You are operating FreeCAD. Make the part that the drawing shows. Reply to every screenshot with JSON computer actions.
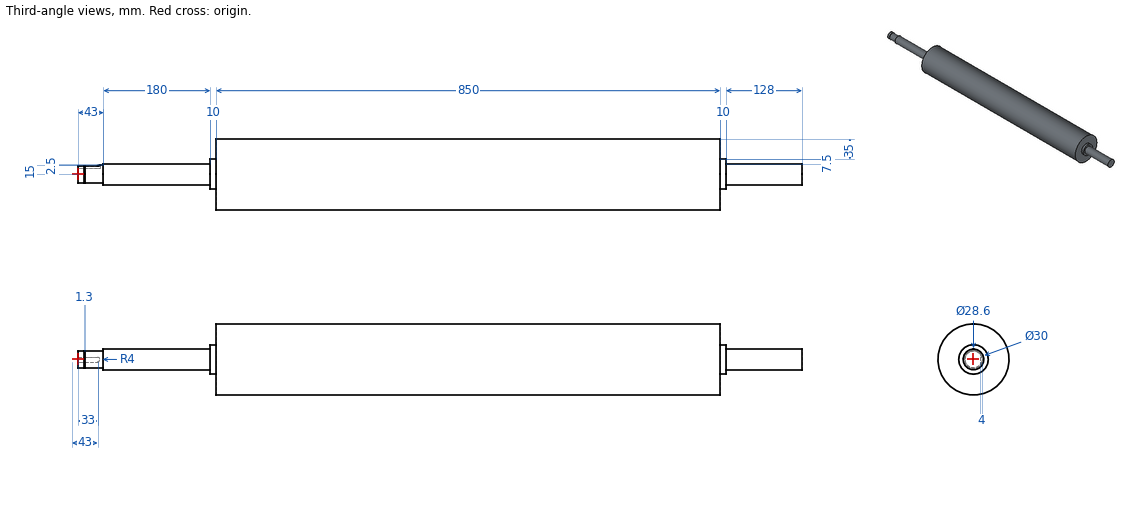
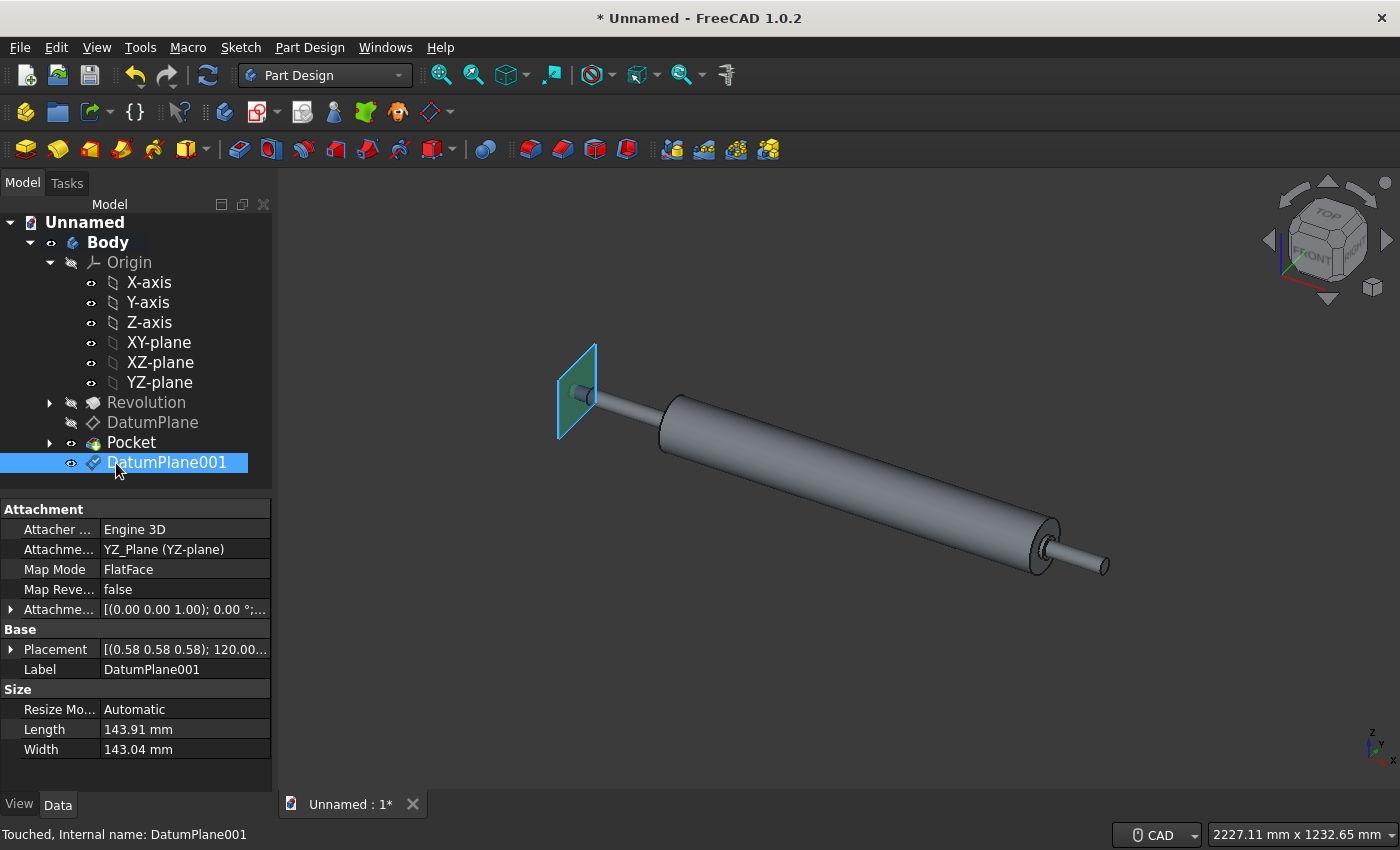
{"action": "left_click", "coordinate": [258, 112]}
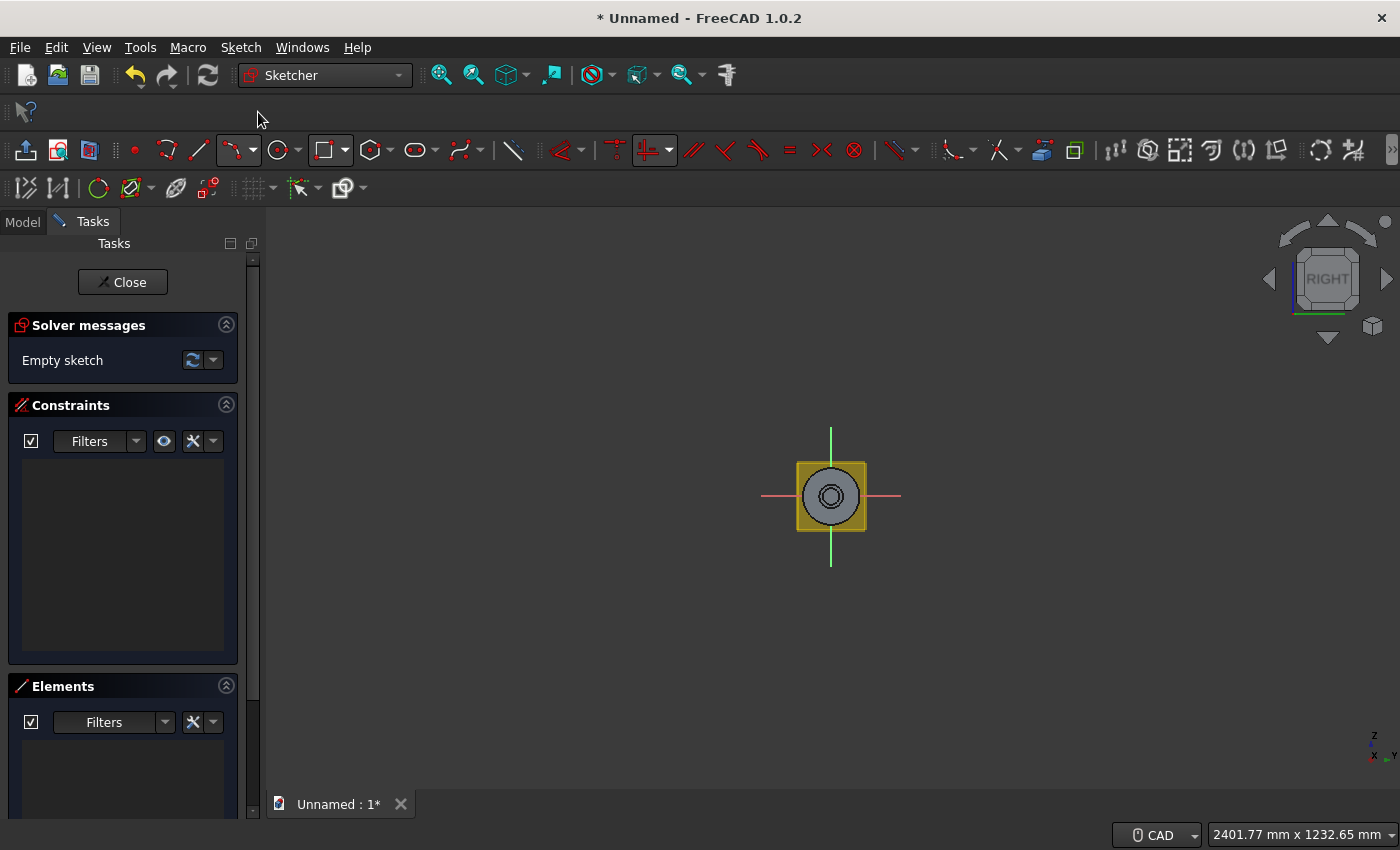
{"action": "left_click", "coordinate": [90, 150]}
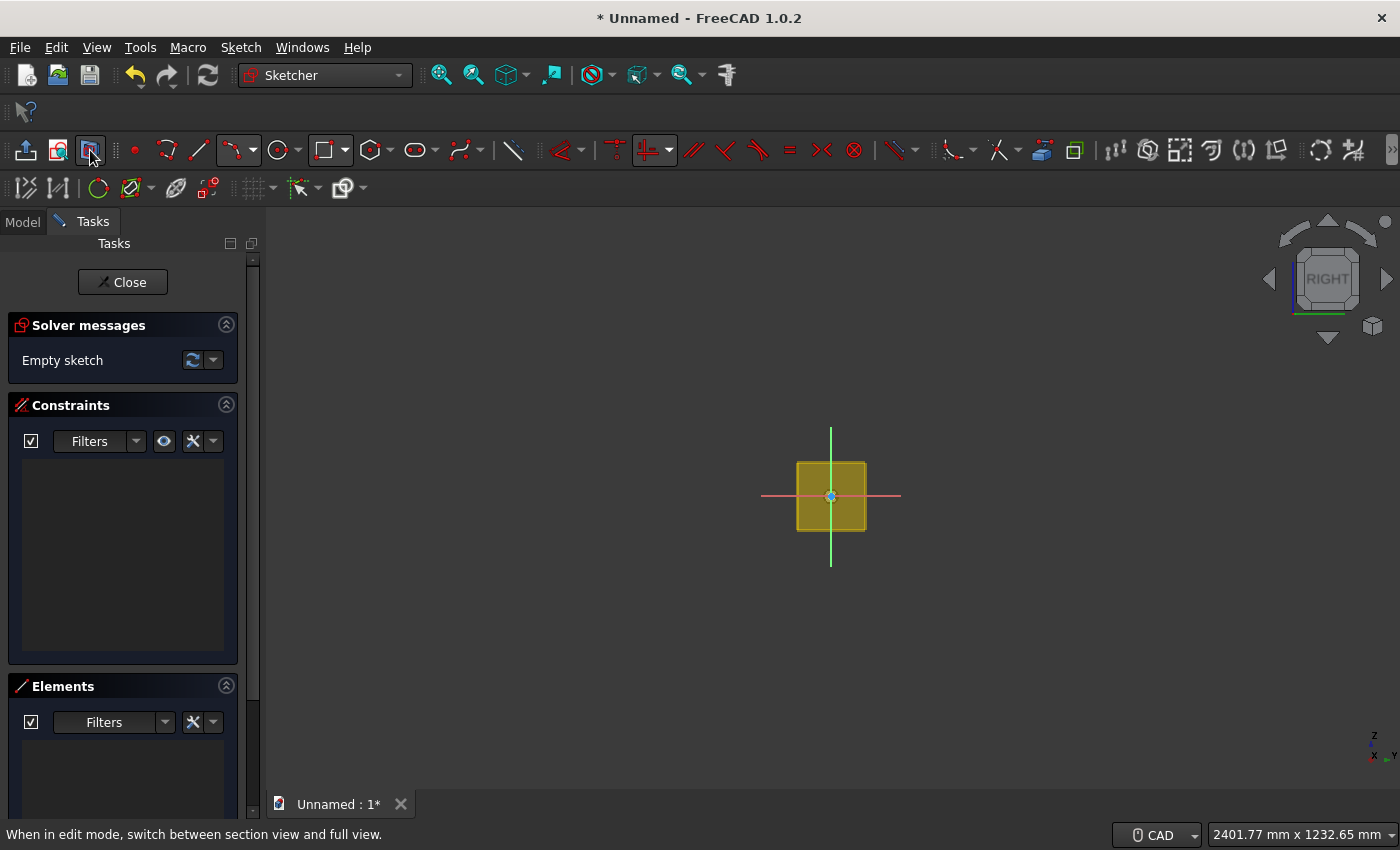
{"action": "scroll", "coordinate": [835, 496], "scroll_direction": "up", "scroll_amount": 15}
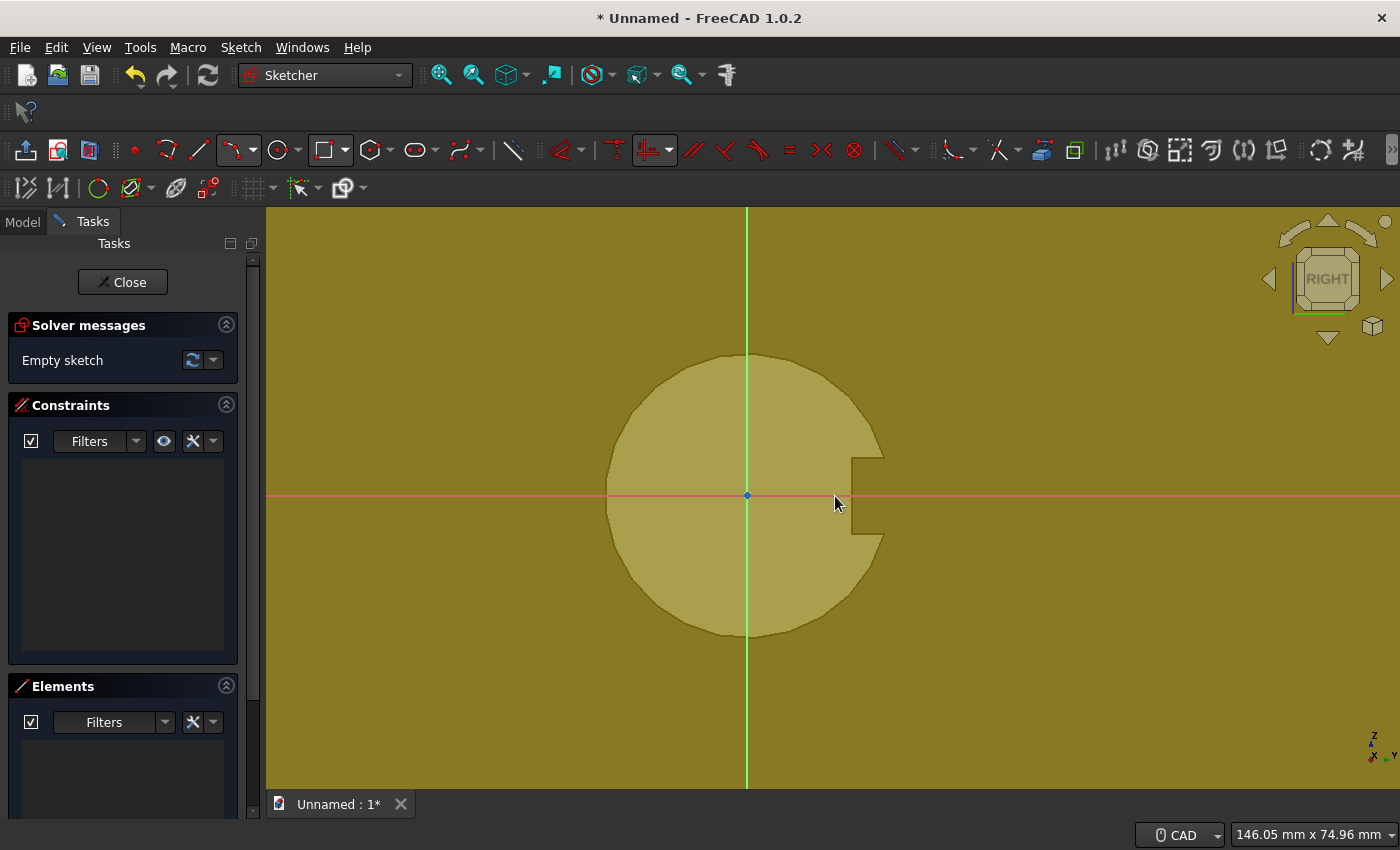
{"action": "left_click", "coordinate": [278, 150]}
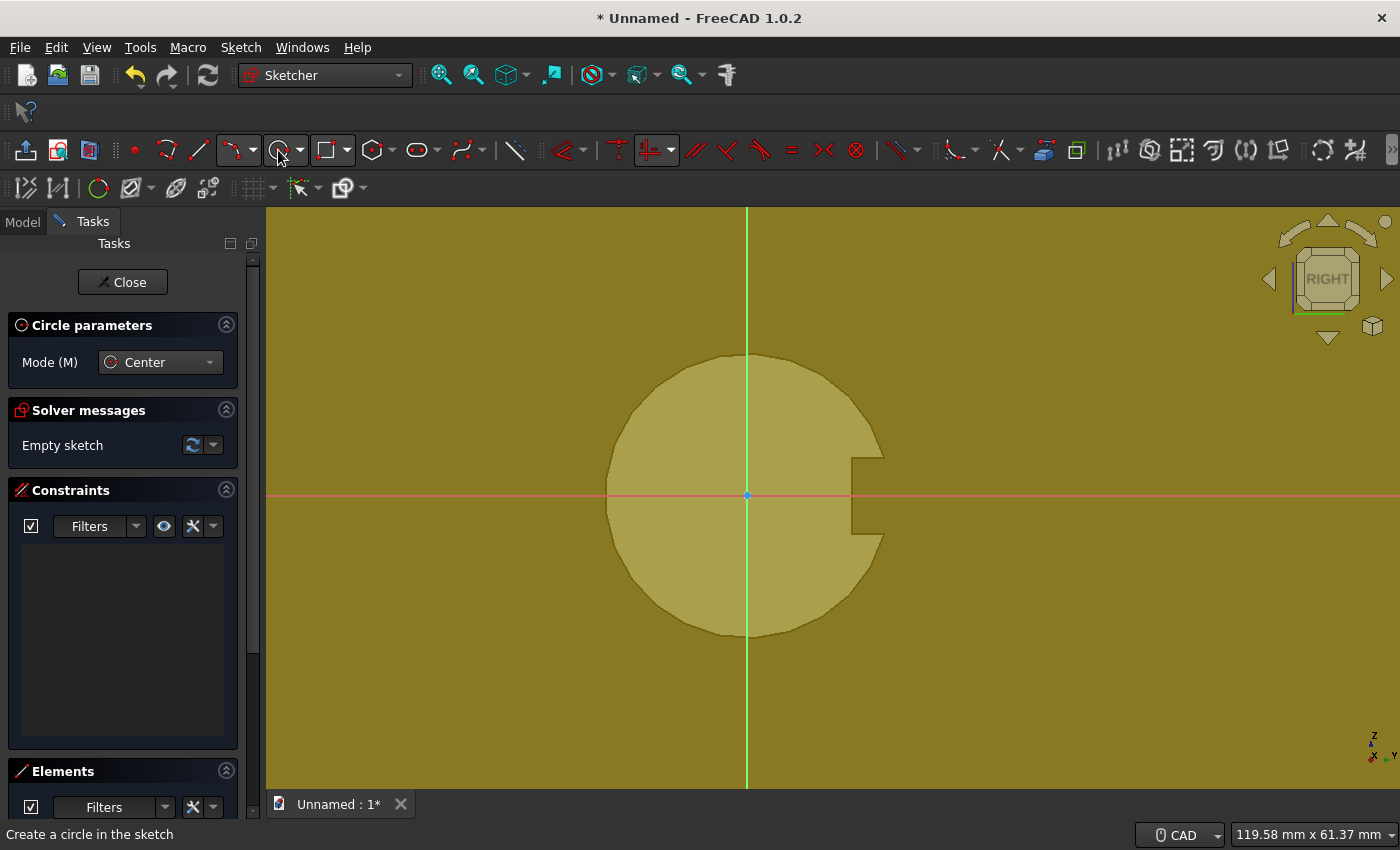
{"action": "left_click", "coordinate": [747, 496]}
{"action": "left_click", "coordinate": [848, 395]}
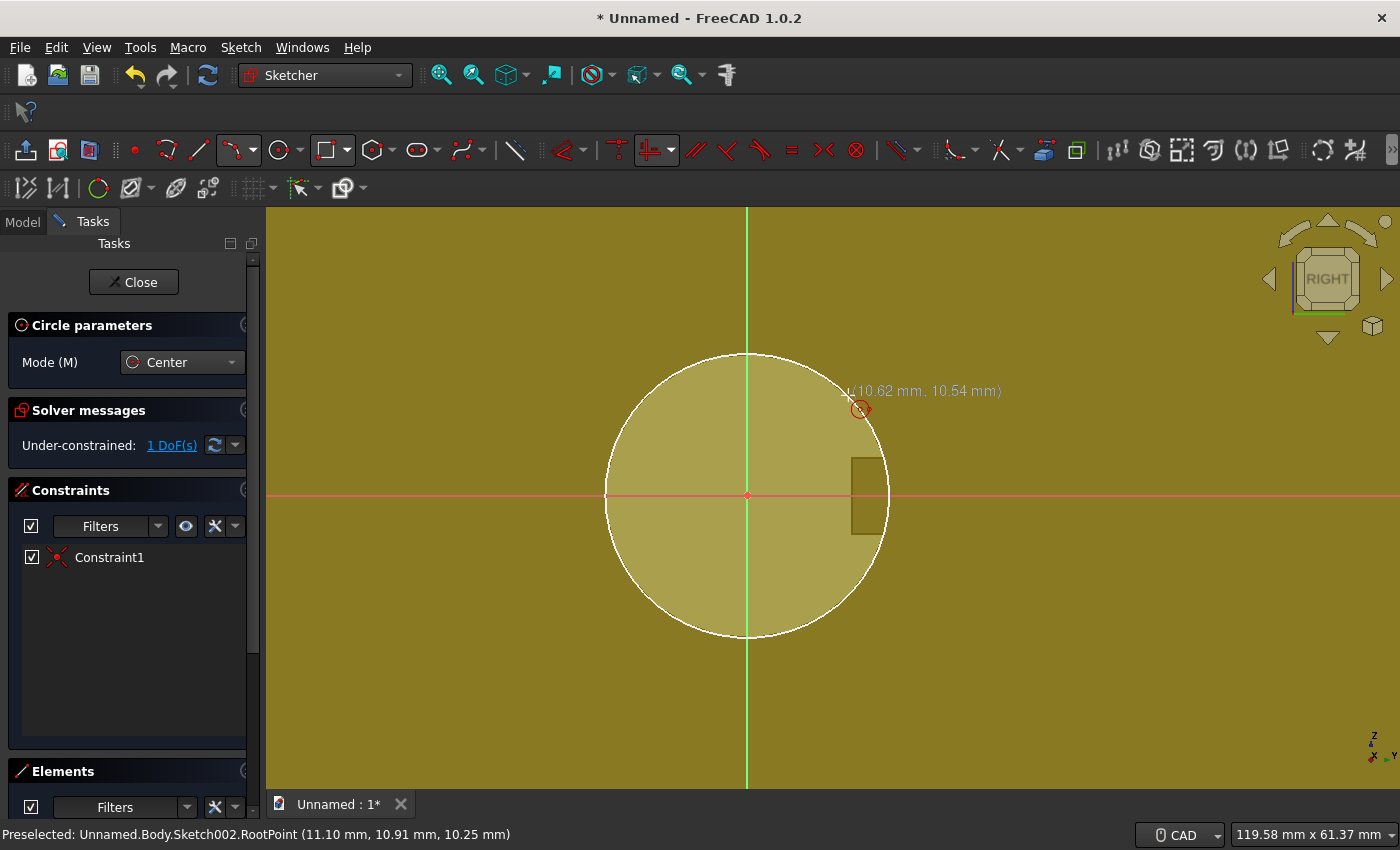
{"action": "left_click", "coordinate": [747, 496]}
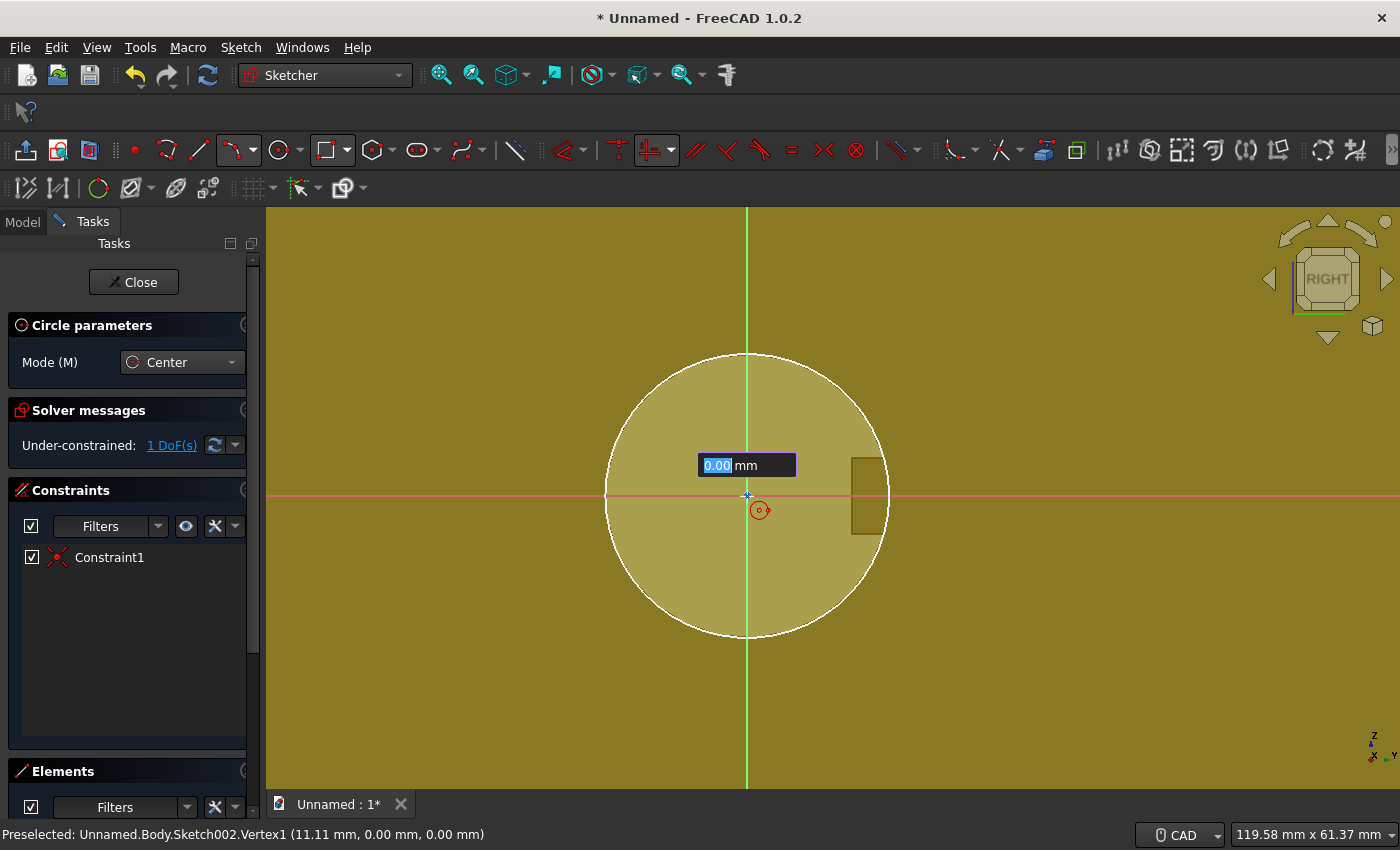
{"action": "scroll", "coordinate": [794, 369], "scroll_direction": "up", "scroll_amount": 5}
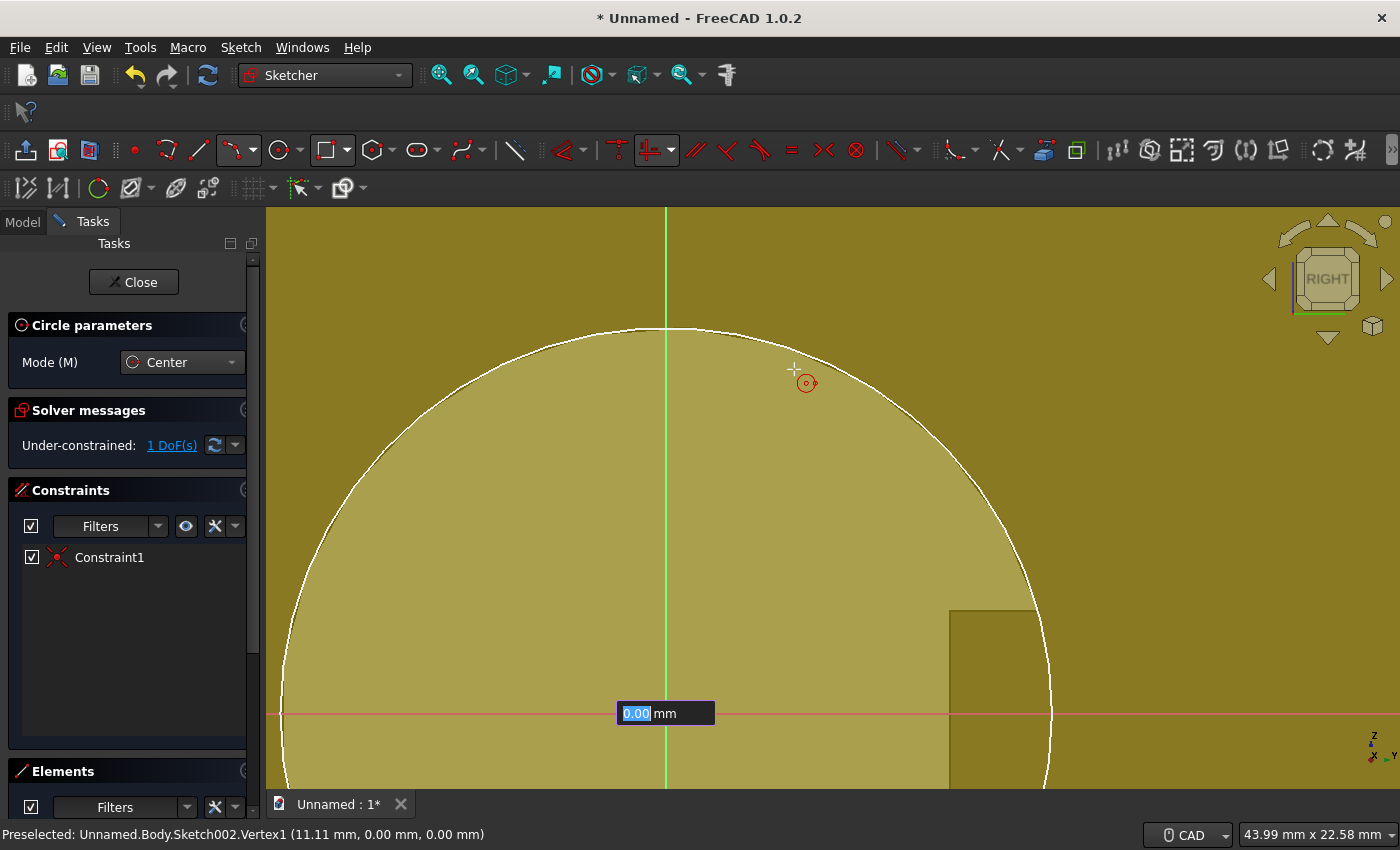
{"action": "left_click", "coordinate": [792, 367]}
{"action": "key", "text": "Escape"}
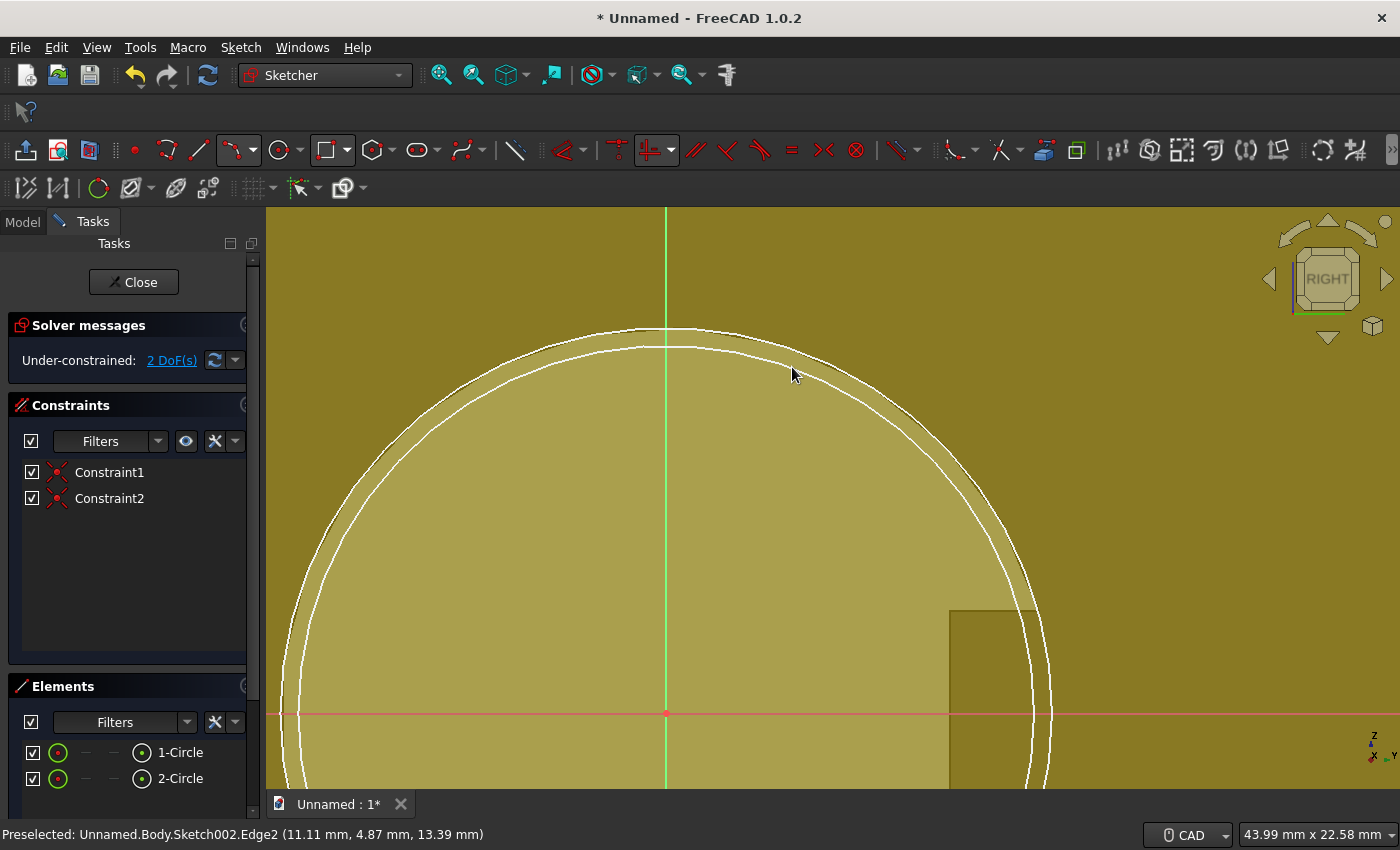
{"action": "left_click", "coordinate": [562, 150]}